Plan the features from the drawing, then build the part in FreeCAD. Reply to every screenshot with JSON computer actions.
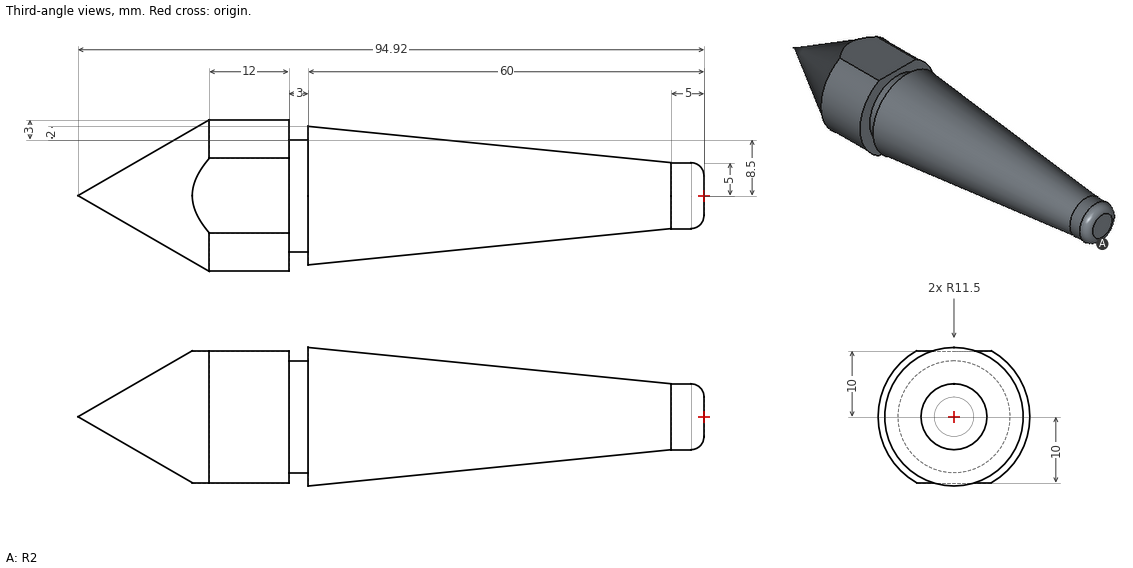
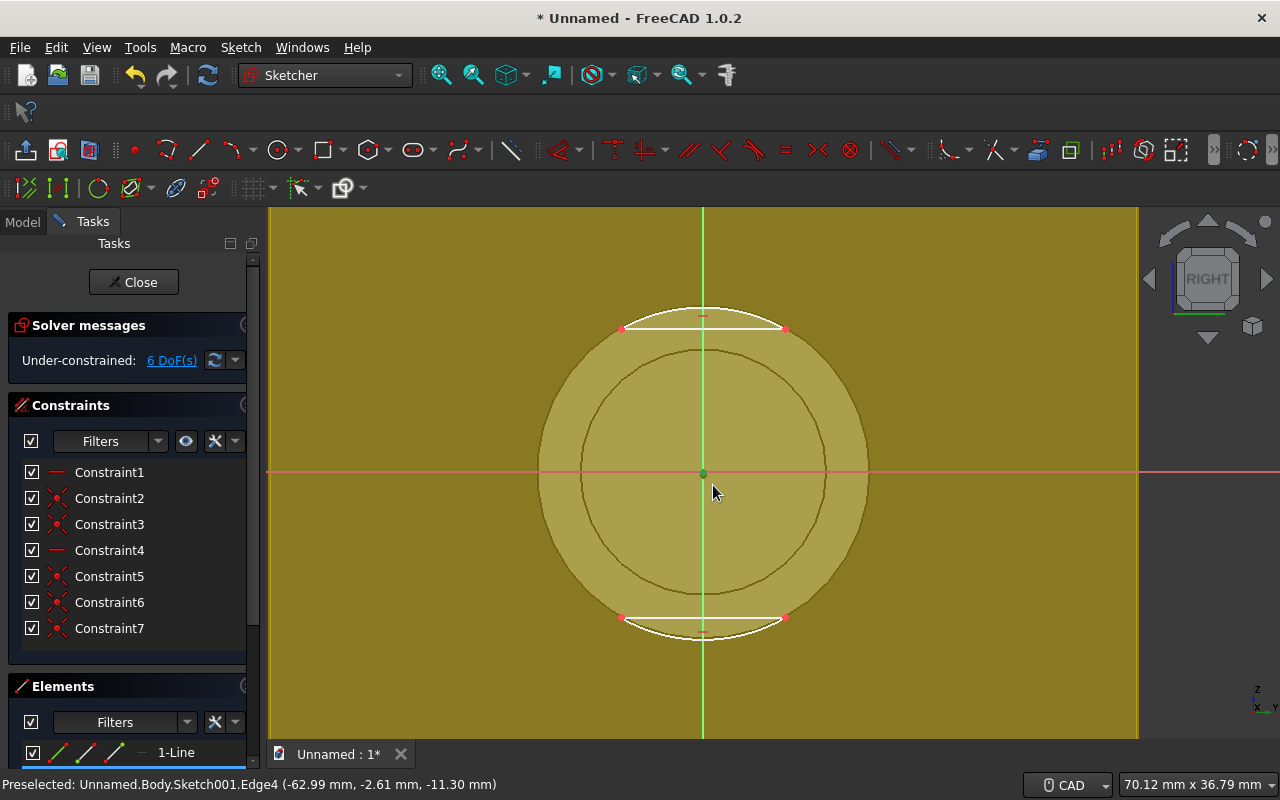
{"action": "left_click", "coordinate": [614, 150]}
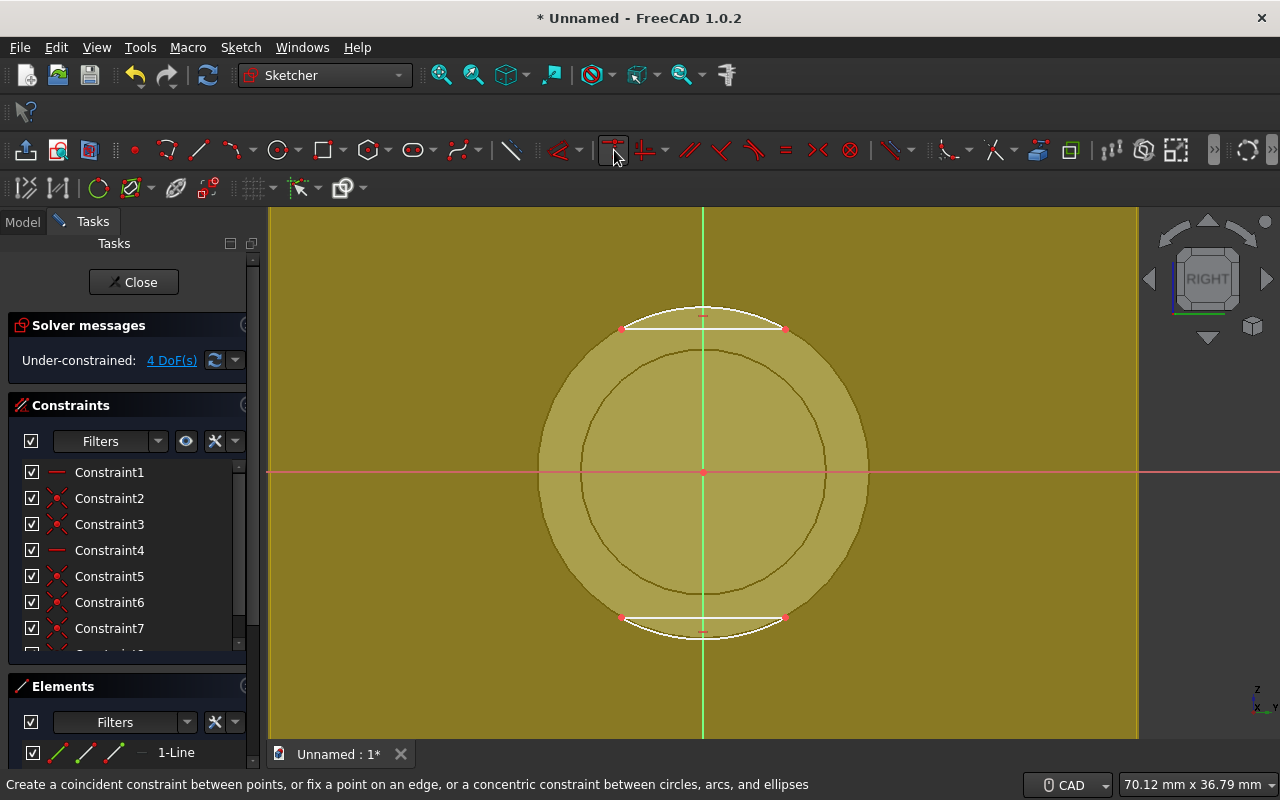
{"action": "left_click", "coordinate": [737, 311]}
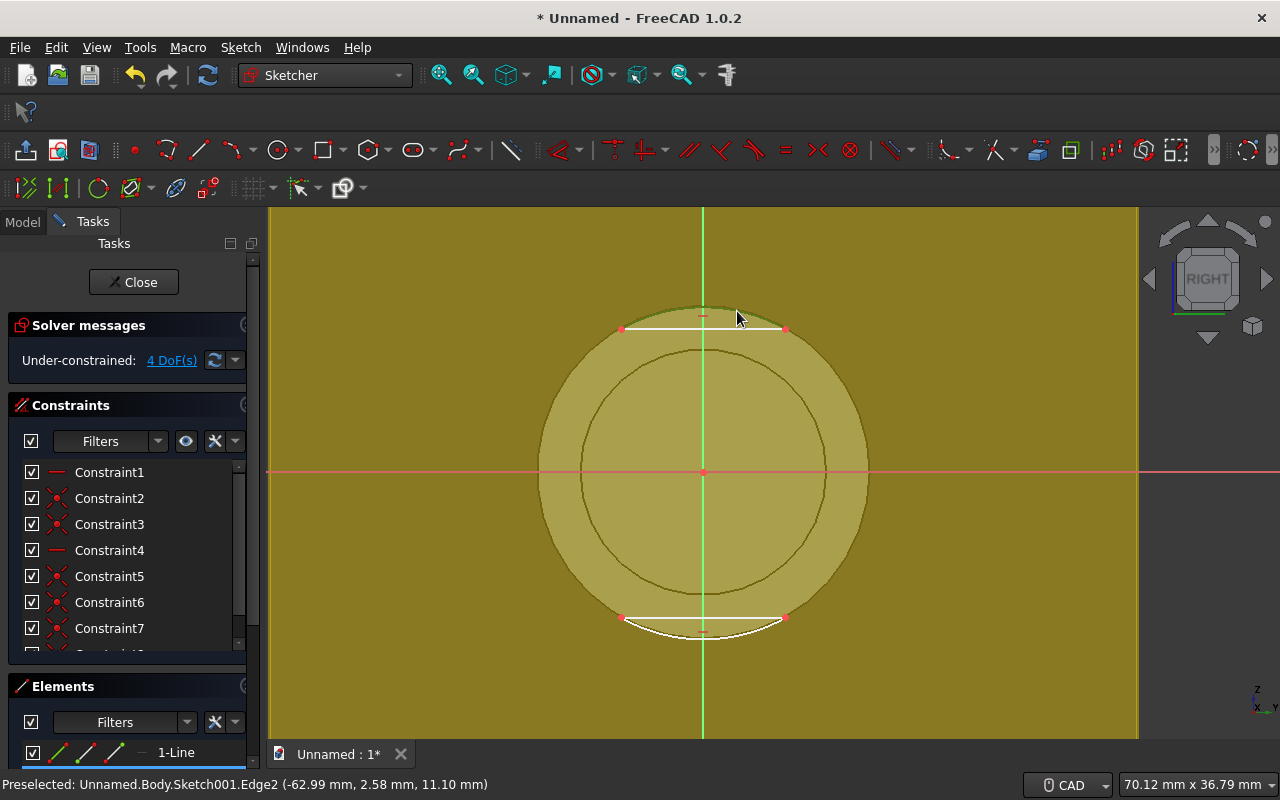
{"action": "left_click", "coordinate": [669, 636]}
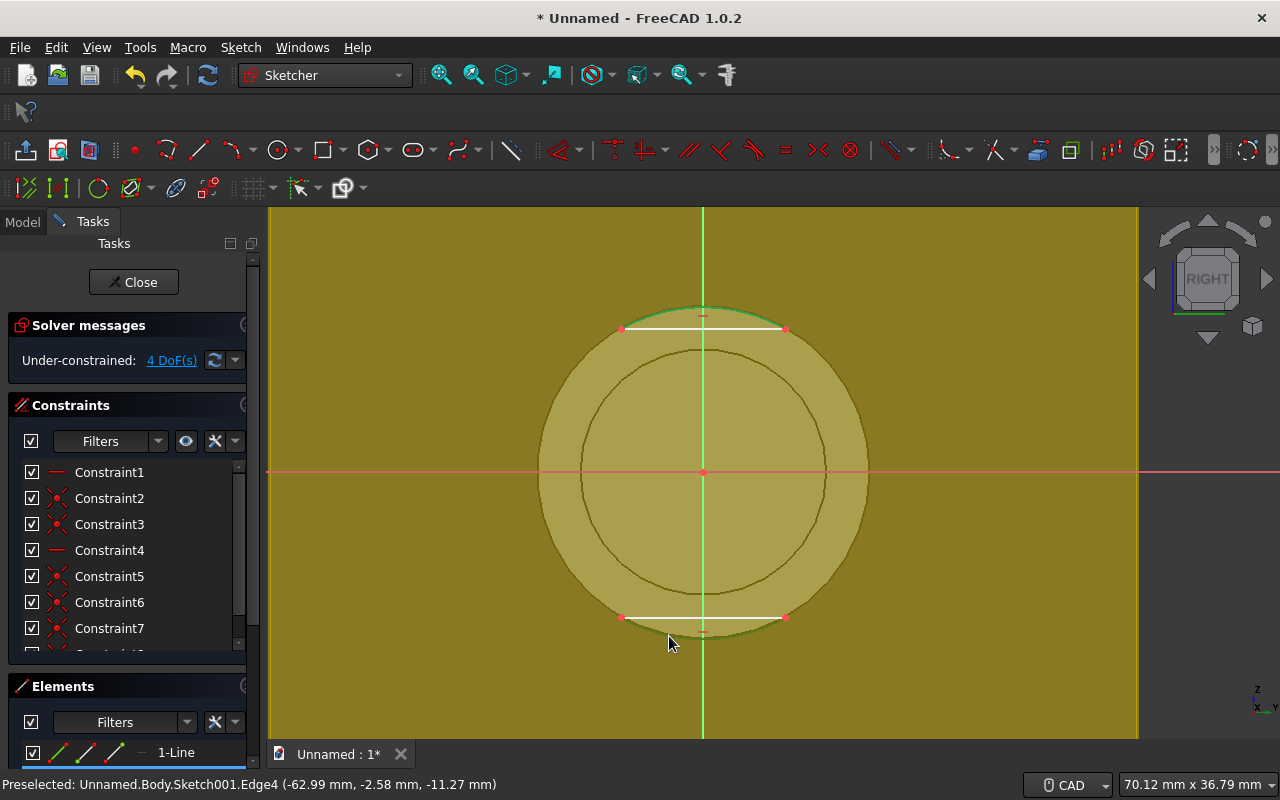
{"action": "left_click", "coordinate": [786, 150]}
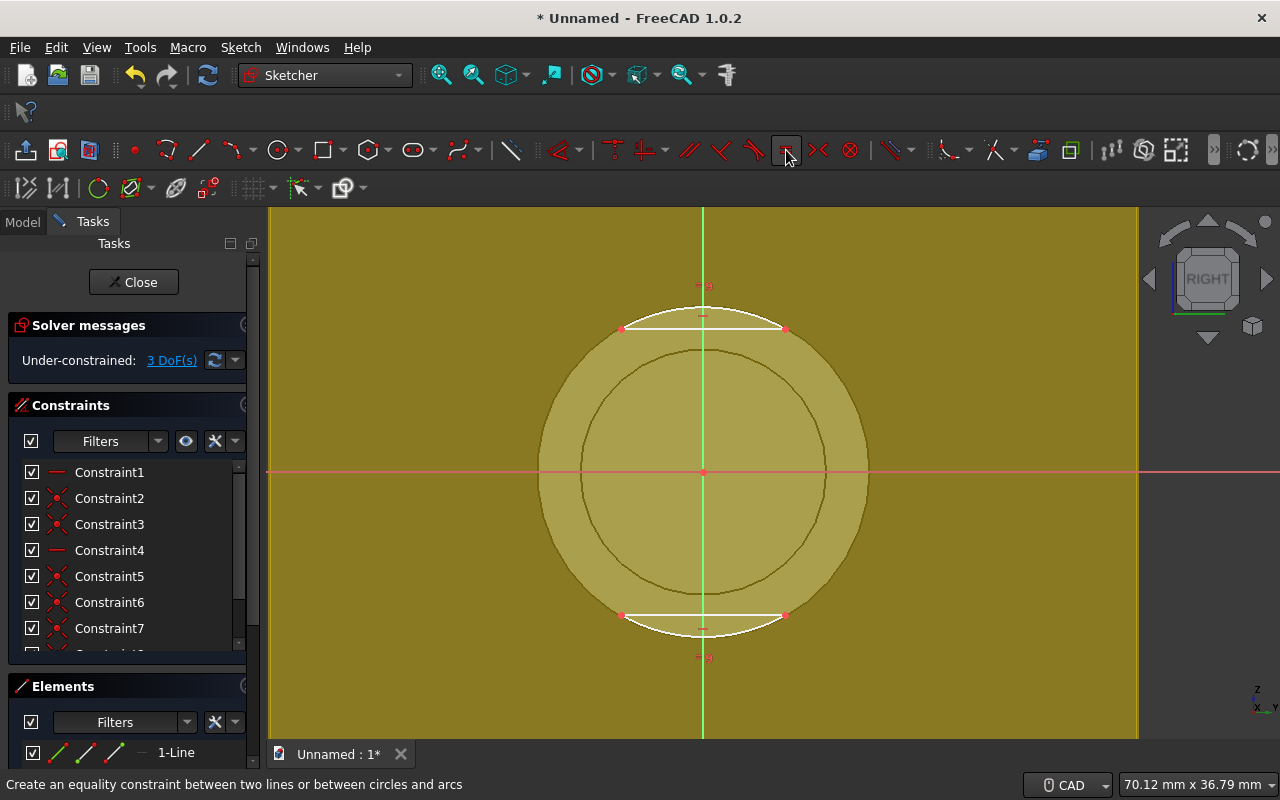
{"action": "left_click", "coordinate": [558, 150]}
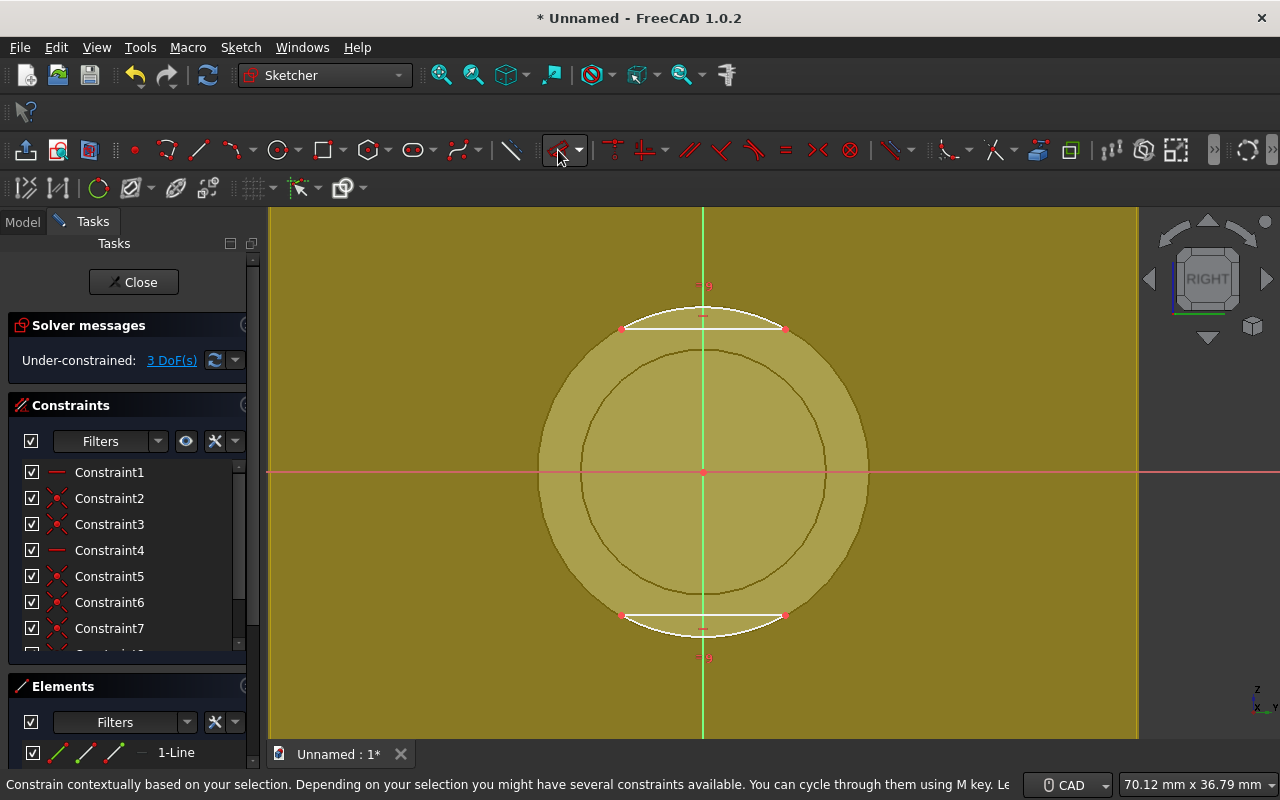
{"action": "left_click", "coordinate": [737, 311]}
{"action": "left_click", "coordinate": [744, 280]}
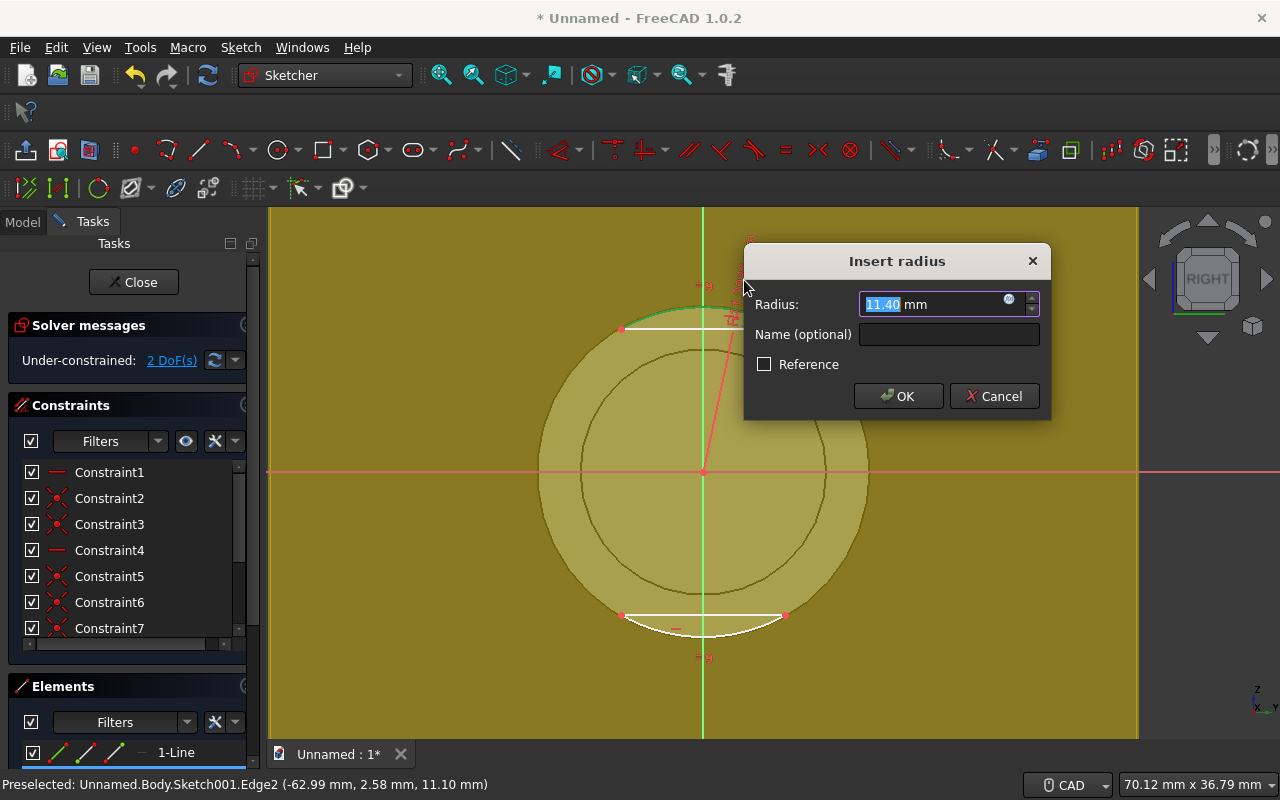
{"action": "type", "text": "11.5"}
{"action": "key", "text": "Return"}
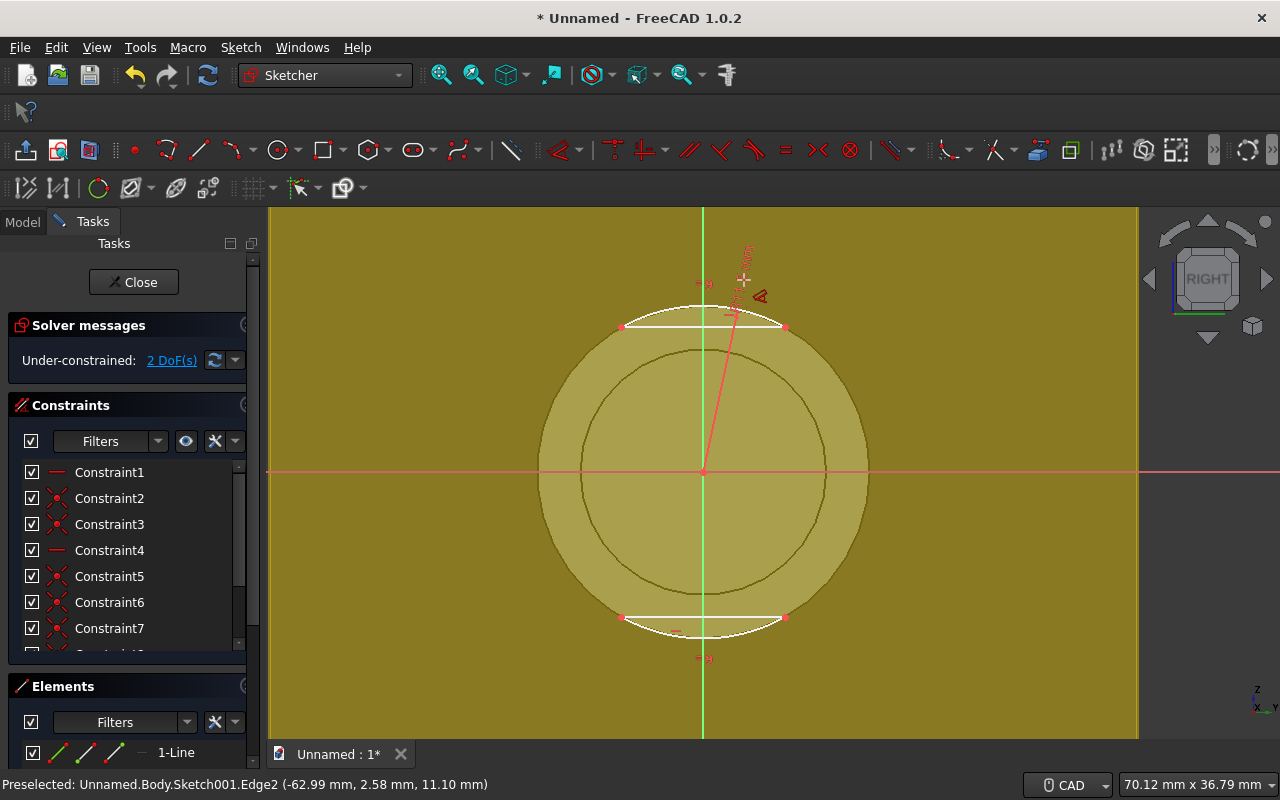
{"action": "left_click", "coordinate": [622, 327]}
{"action": "left_click", "coordinate": [588, 400]}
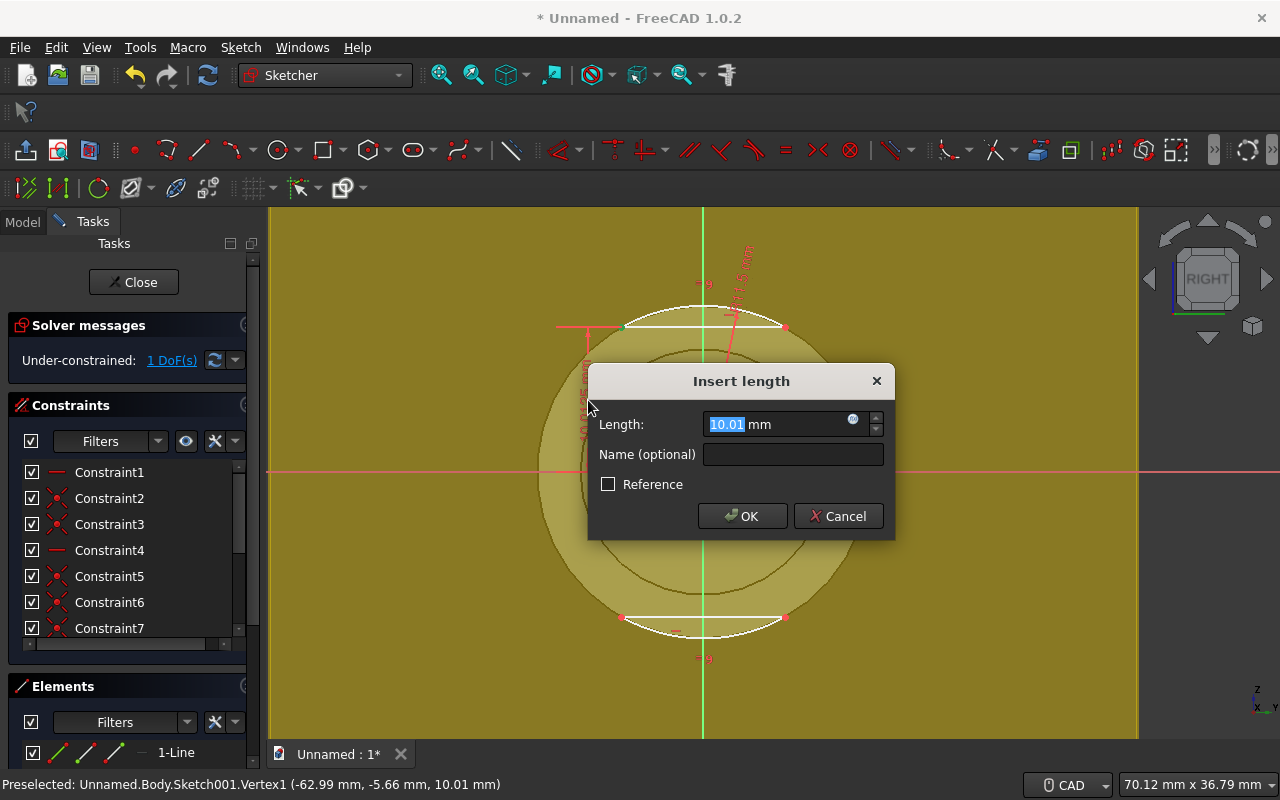
{"action": "type", "text": "10"}
{"action": "key", "text": "Return"}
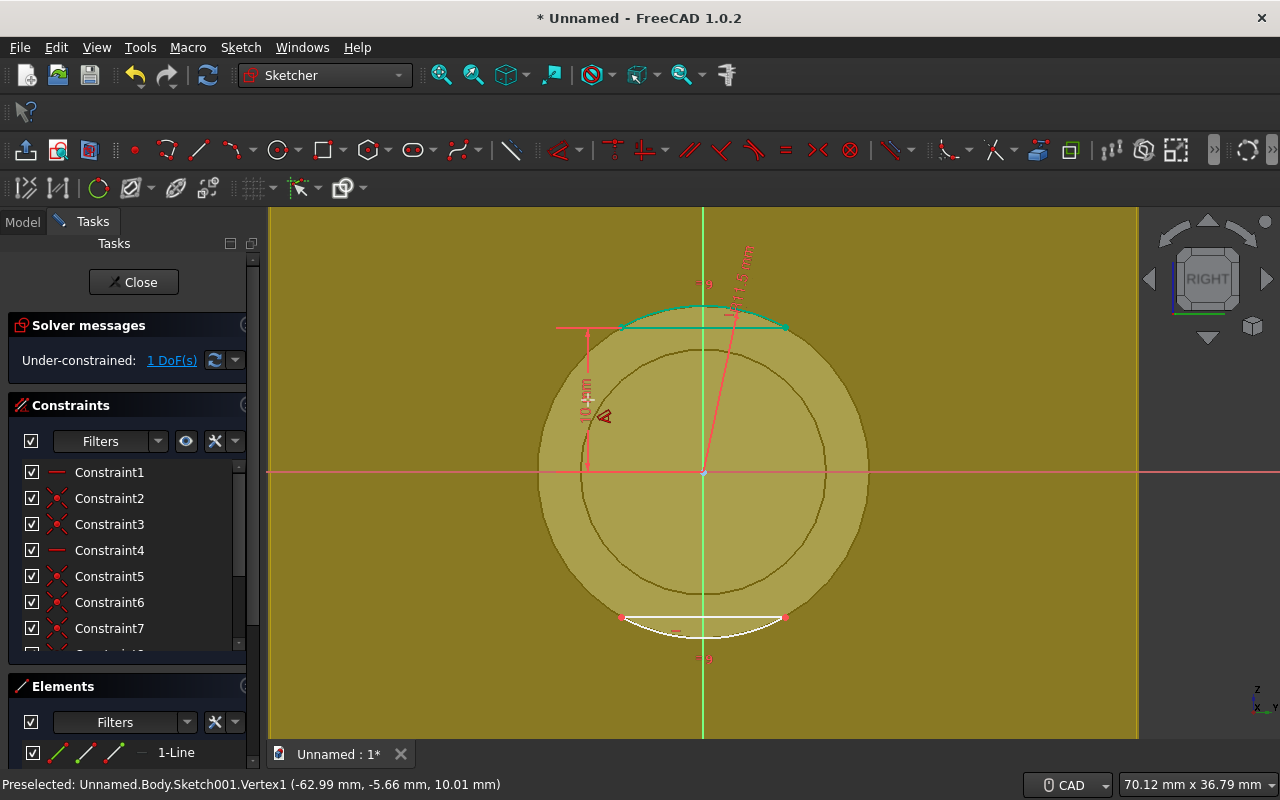
{"action": "left_click", "coordinate": [785, 617]}
{"action": "left_click", "coordinate": [819, 545]}